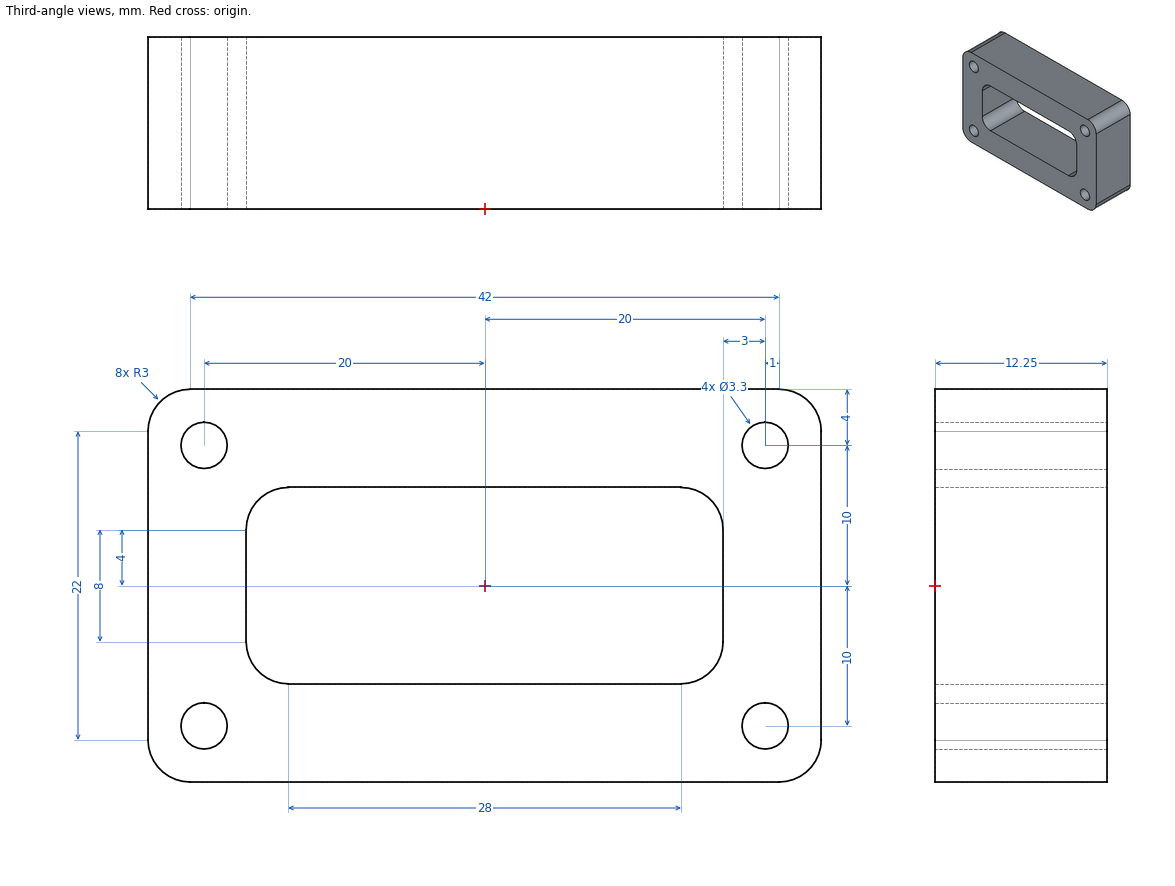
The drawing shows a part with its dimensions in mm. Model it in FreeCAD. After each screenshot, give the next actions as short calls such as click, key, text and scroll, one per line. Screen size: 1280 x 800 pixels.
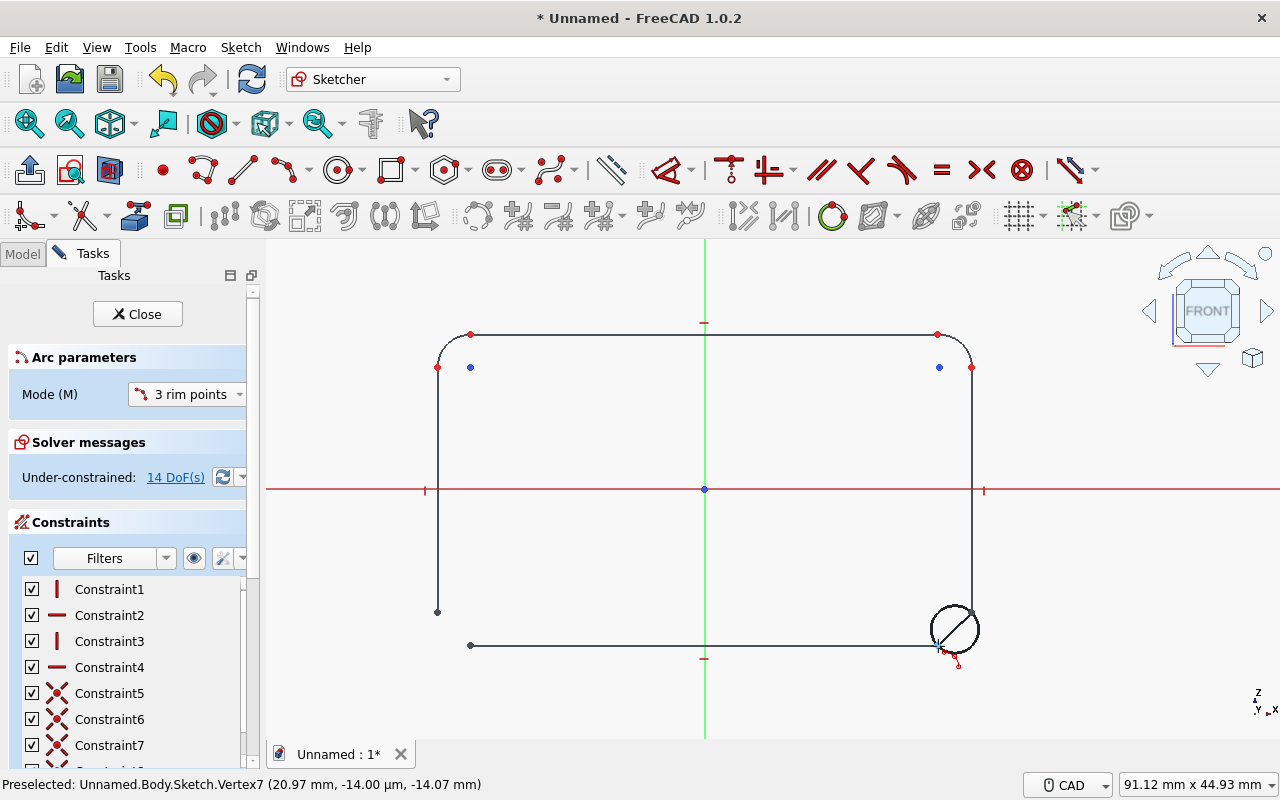
scroll(962, 635, up, 3)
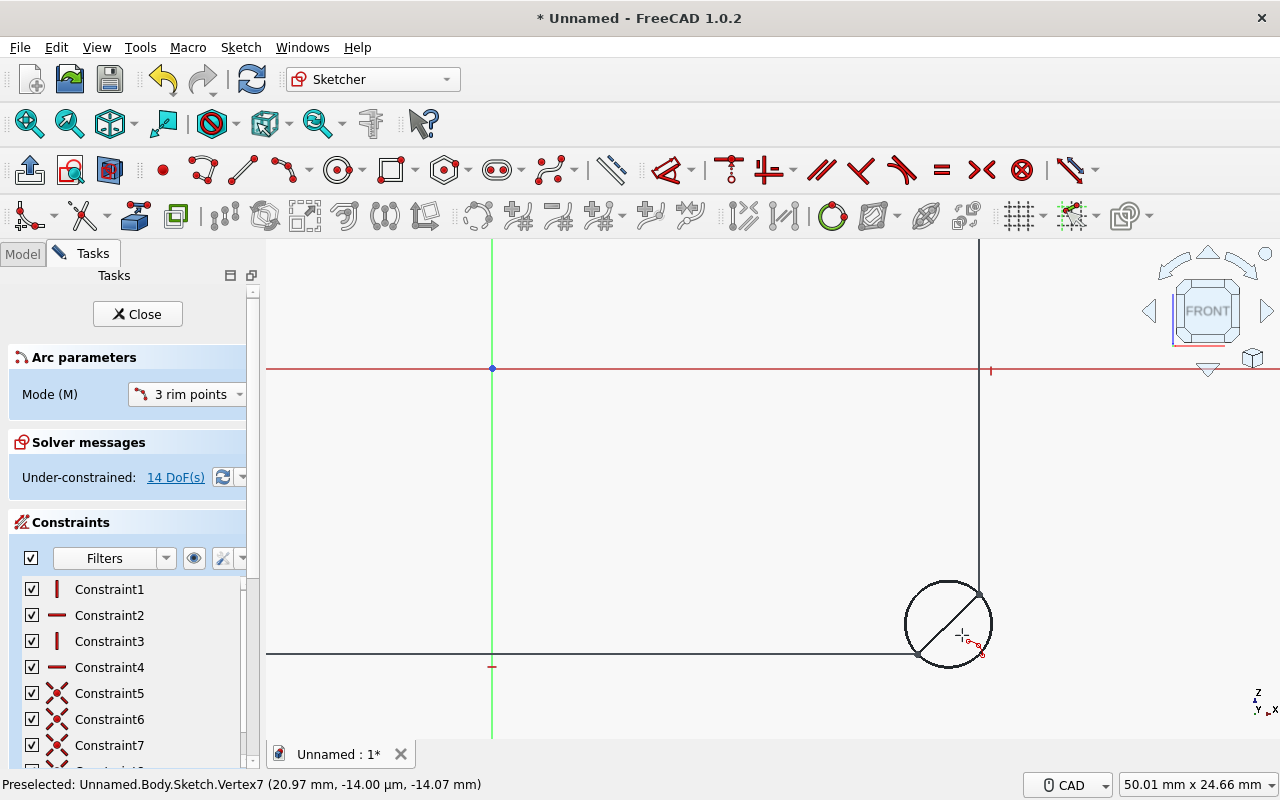
click(961, 635)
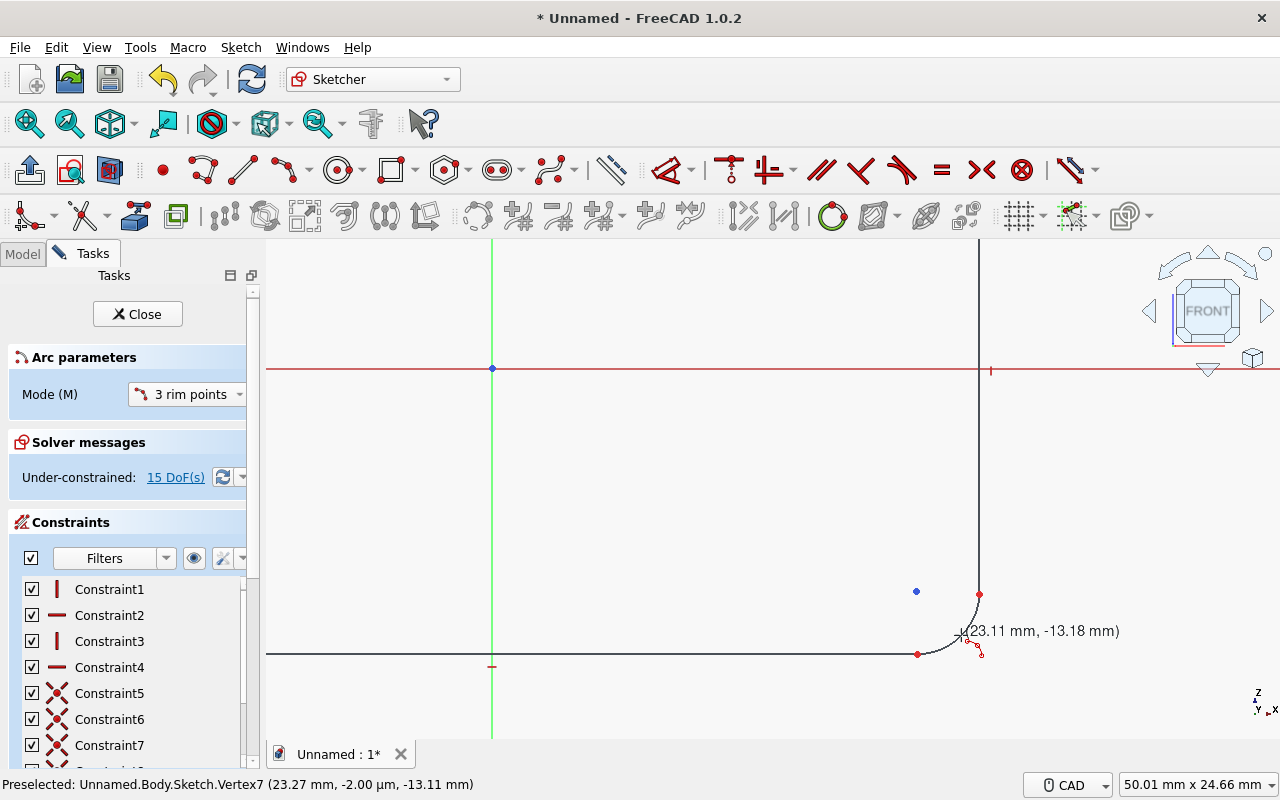
scroll(962, 635, down, 3)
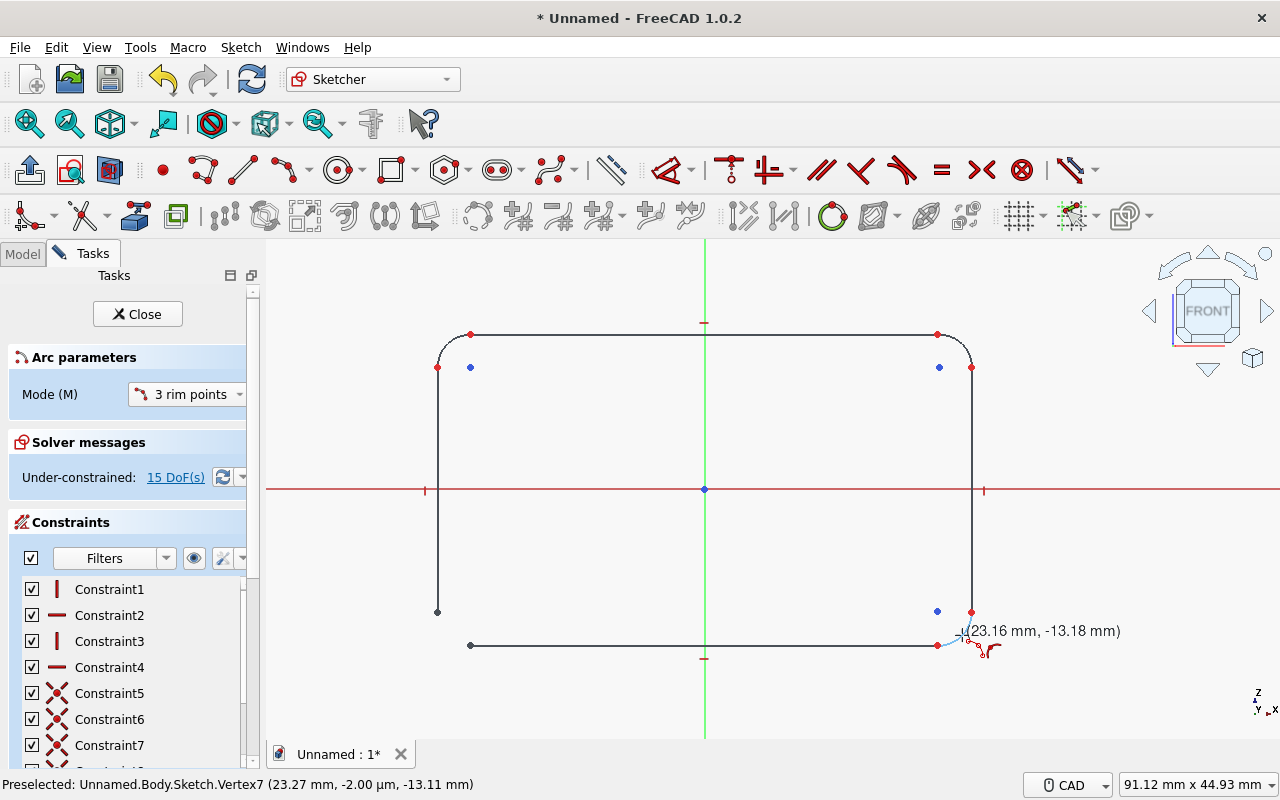
click(471, 646)
click(438, 613)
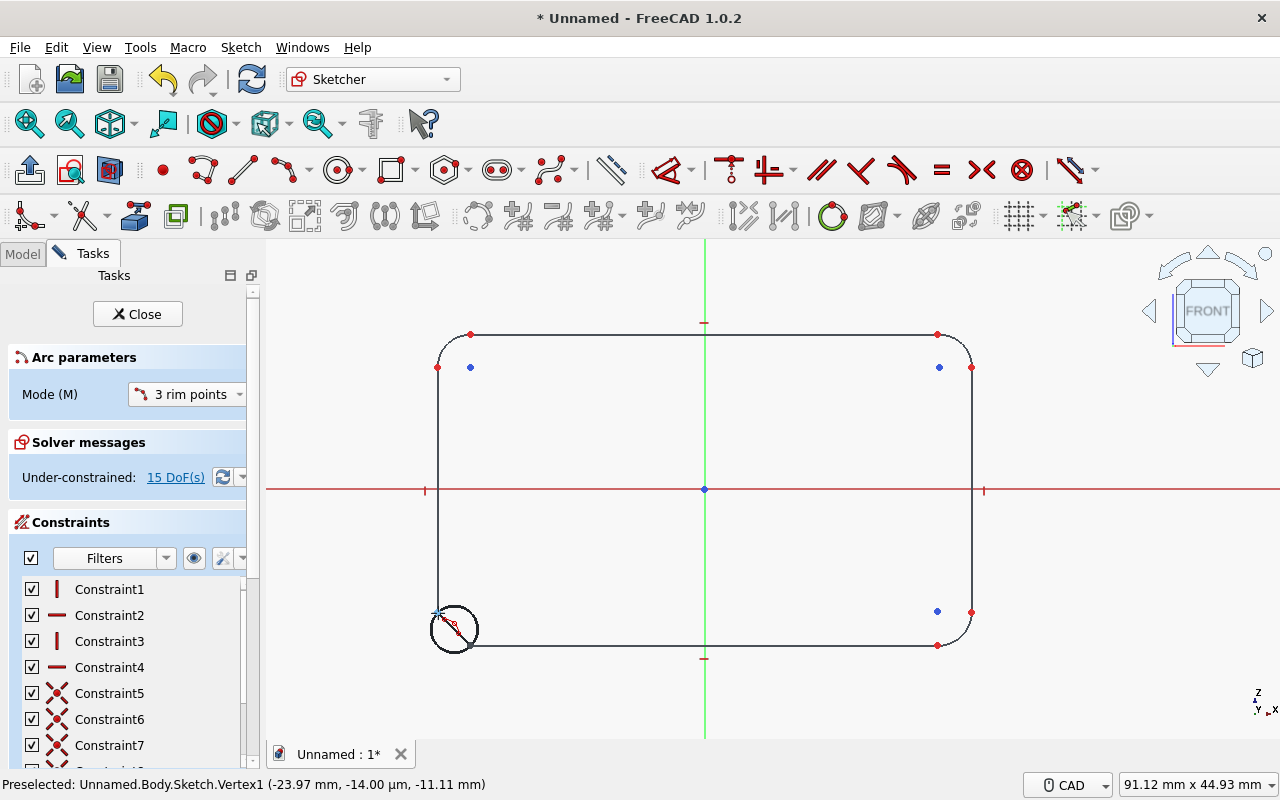
scroll(447, 635, up, 3)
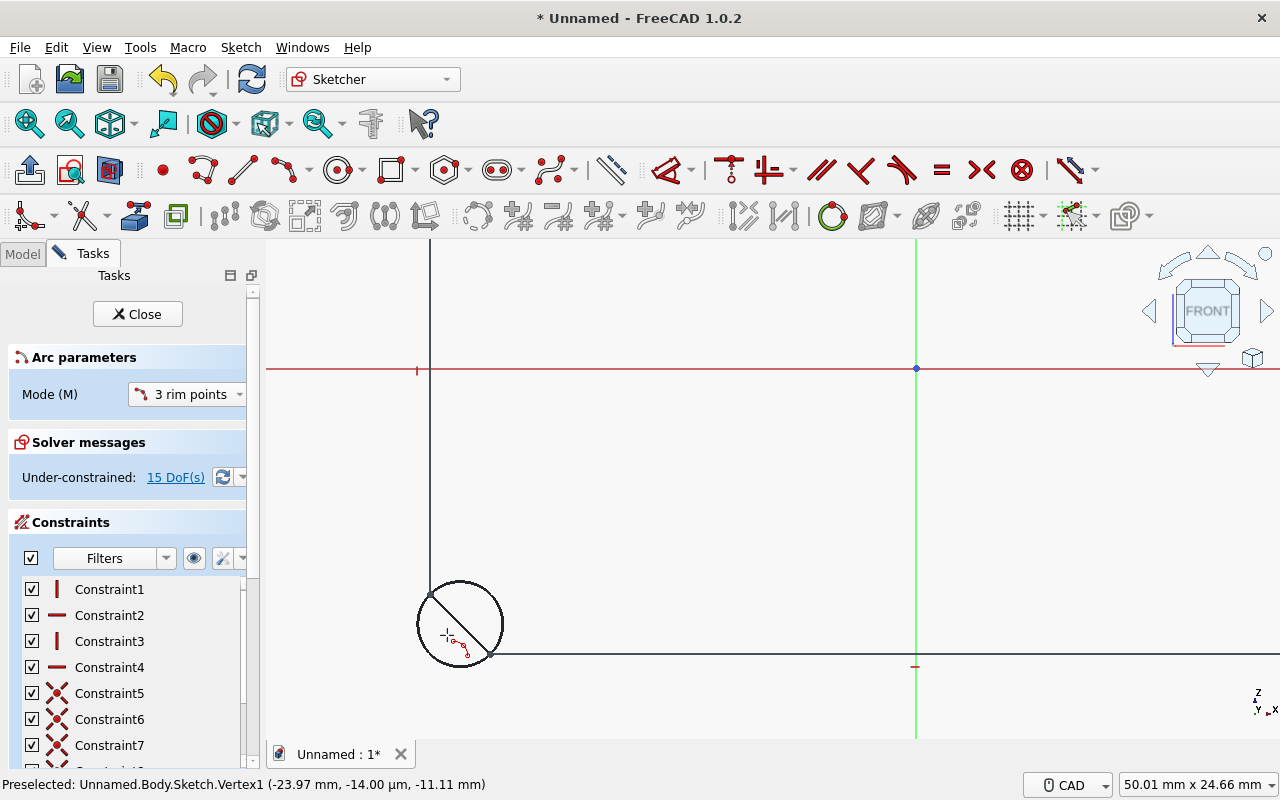
click(447, 635)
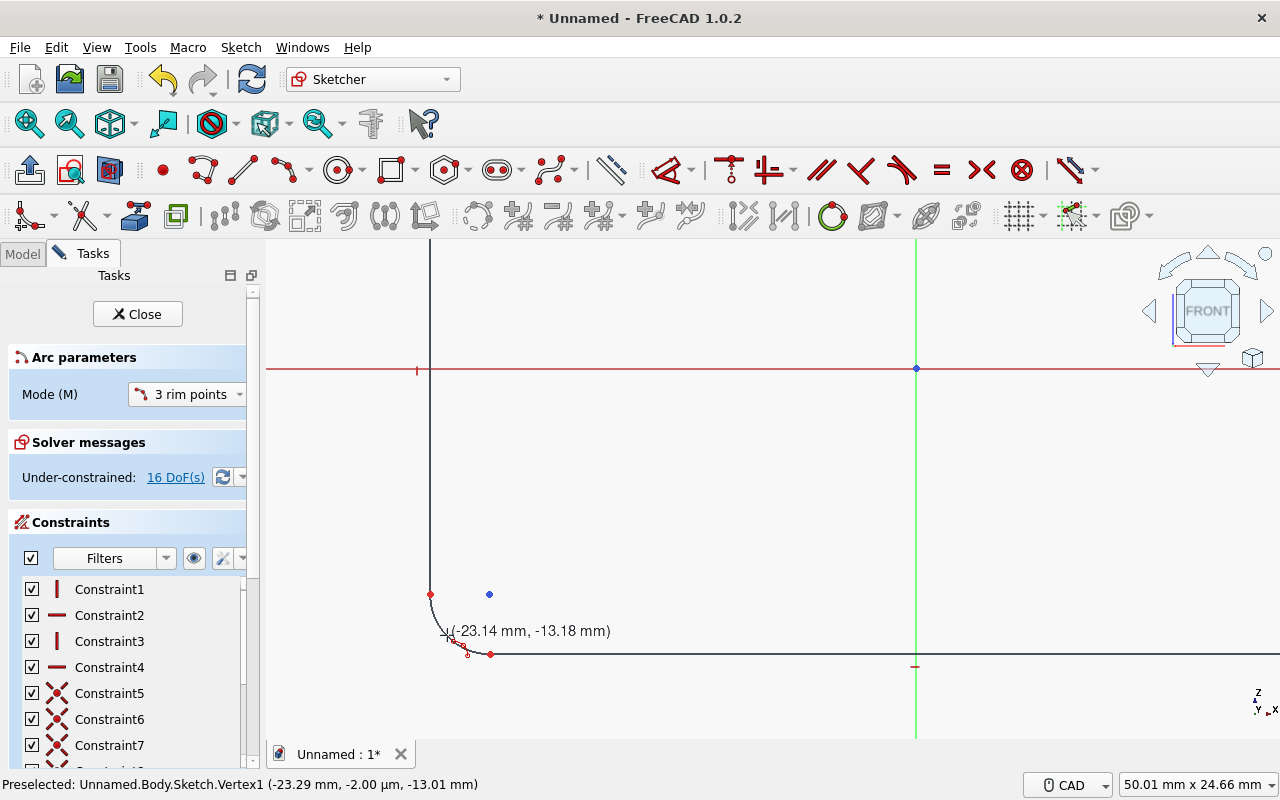
click(244, 170)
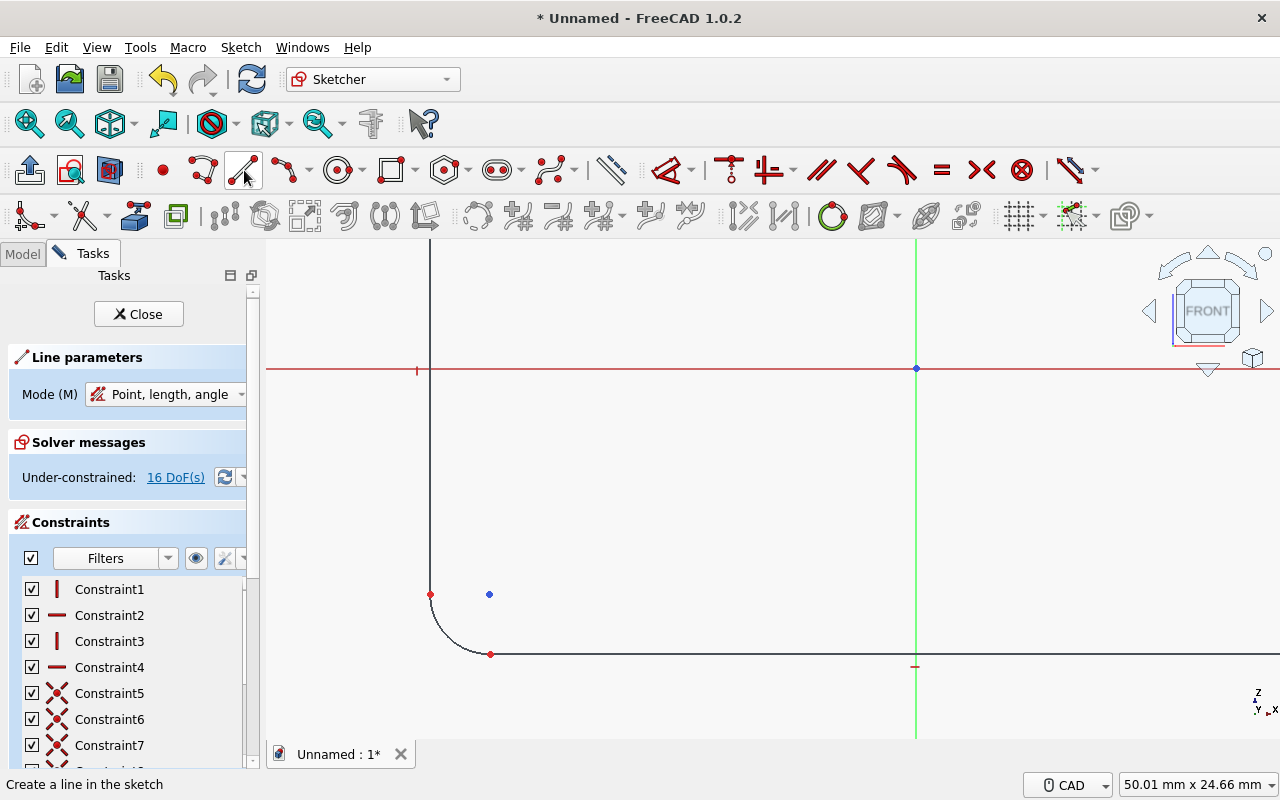
click(572, 288)
click(572, 450)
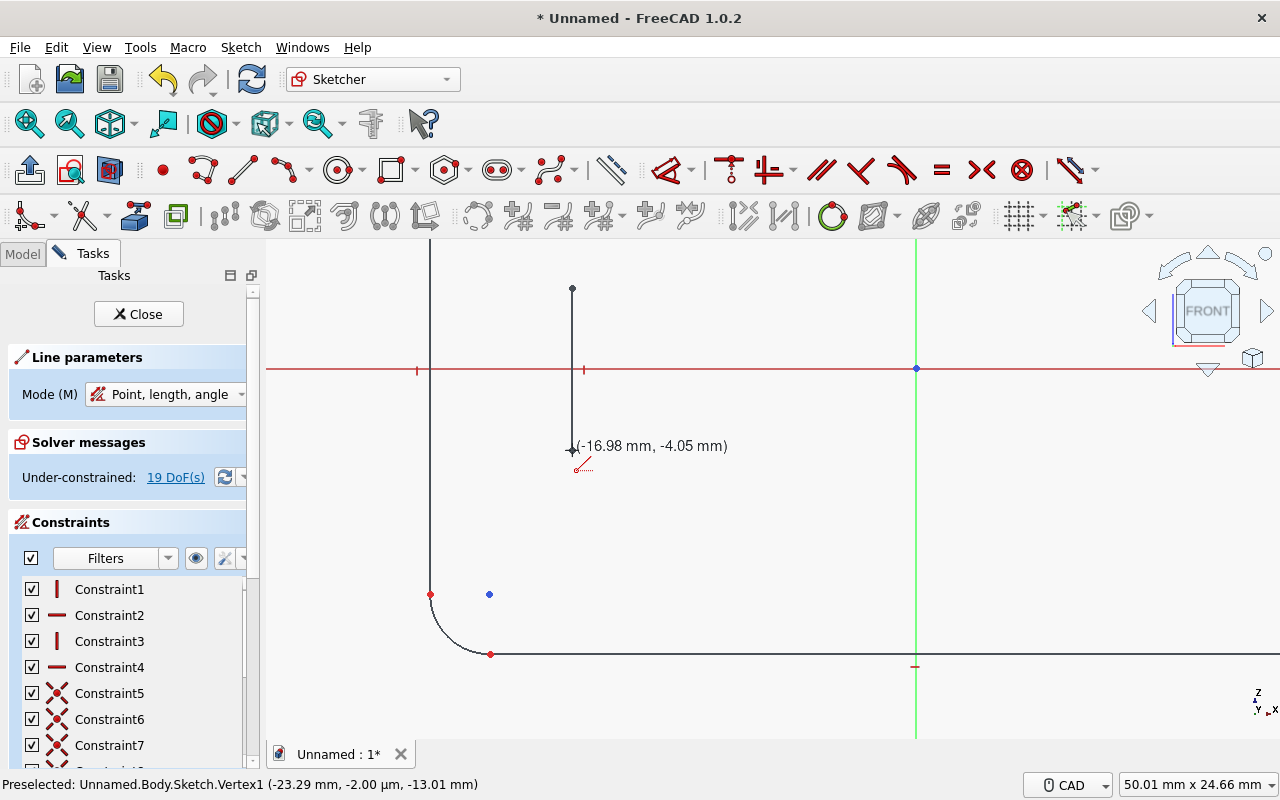
click(632, 511)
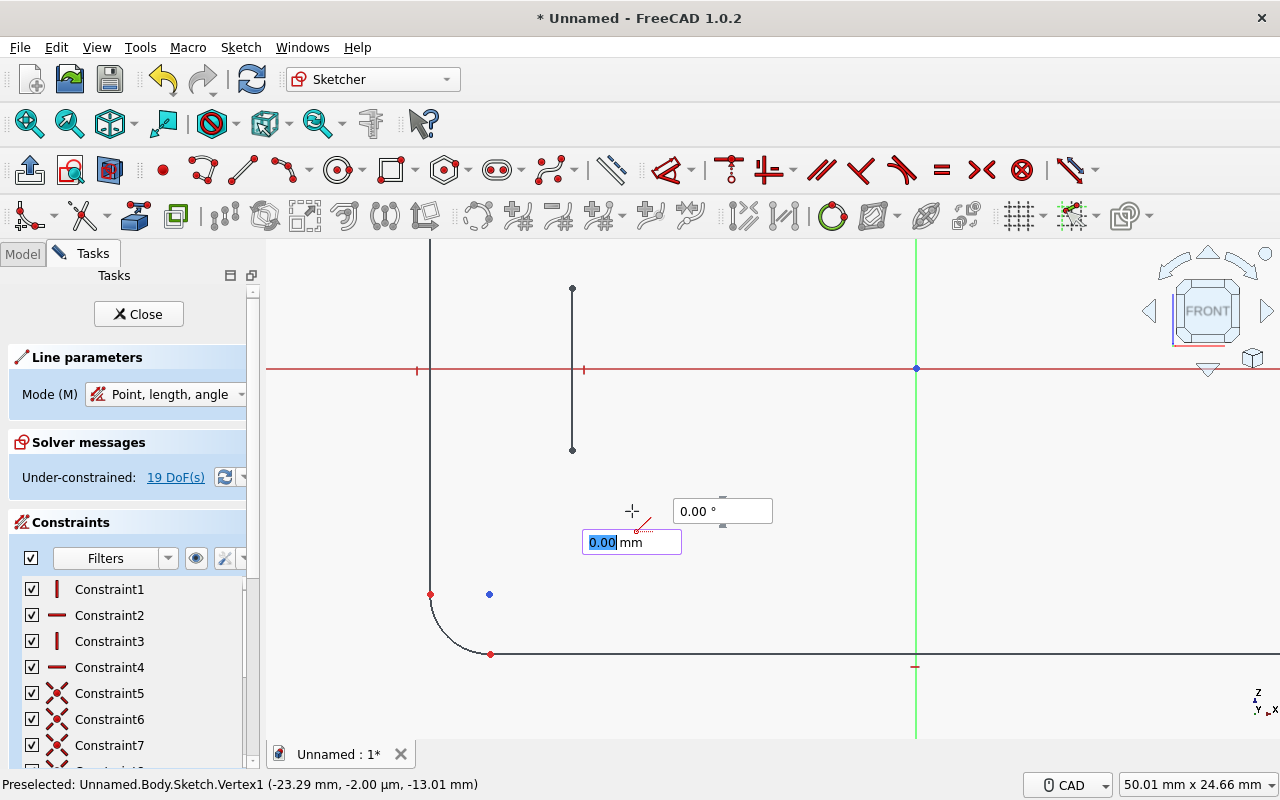
scroll(447, 635, down, 3)